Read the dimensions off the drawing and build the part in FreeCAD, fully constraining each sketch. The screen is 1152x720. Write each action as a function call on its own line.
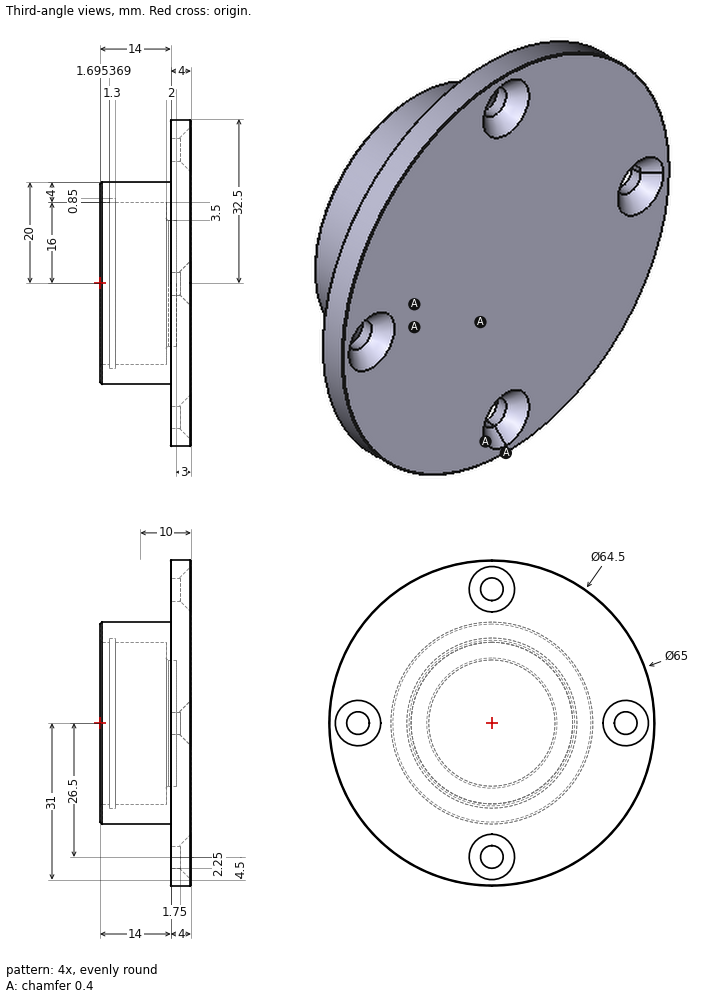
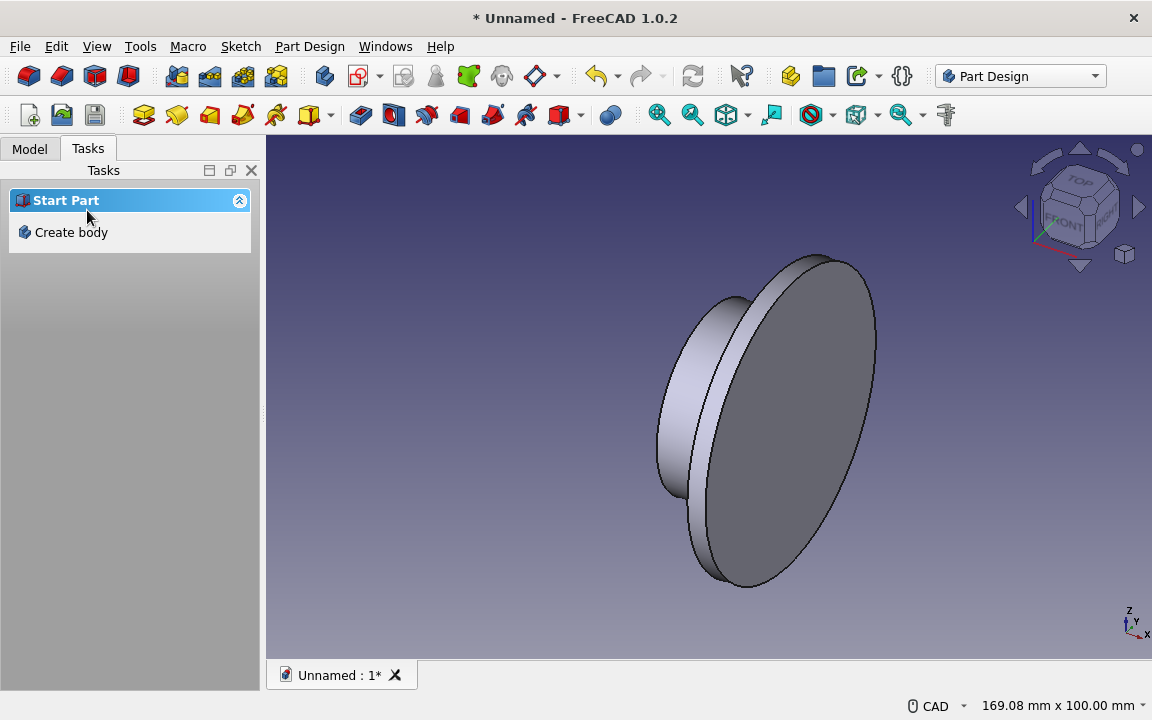
click(358, 76)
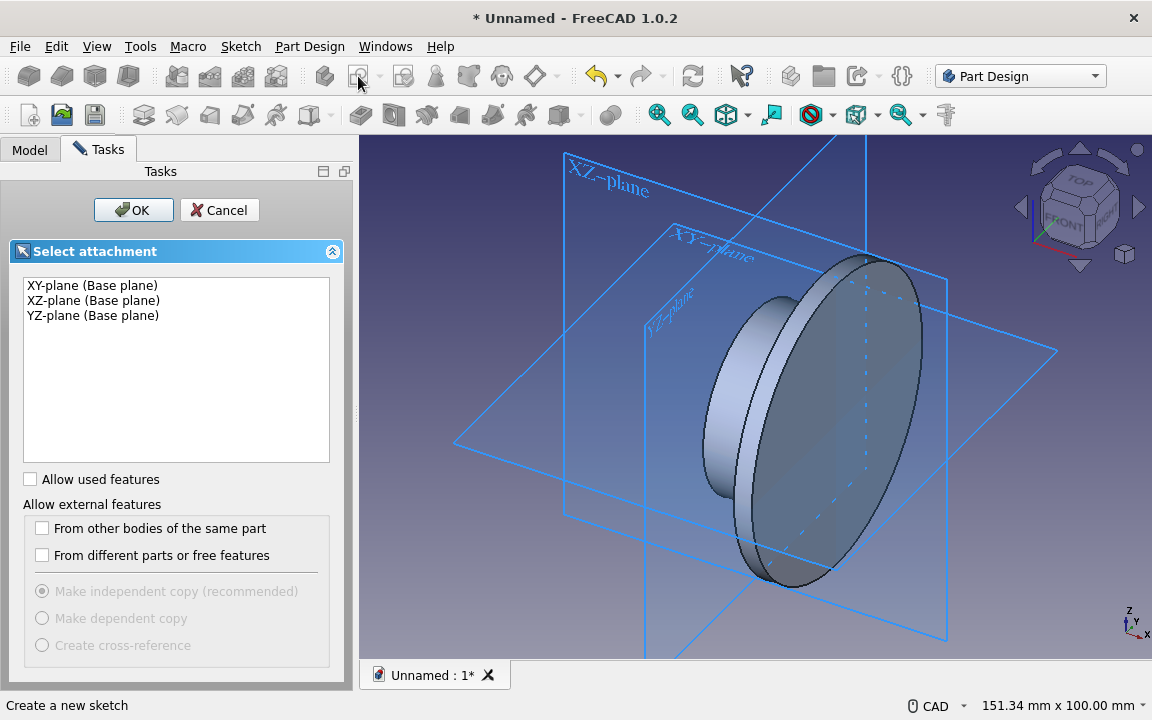
click(84, 300)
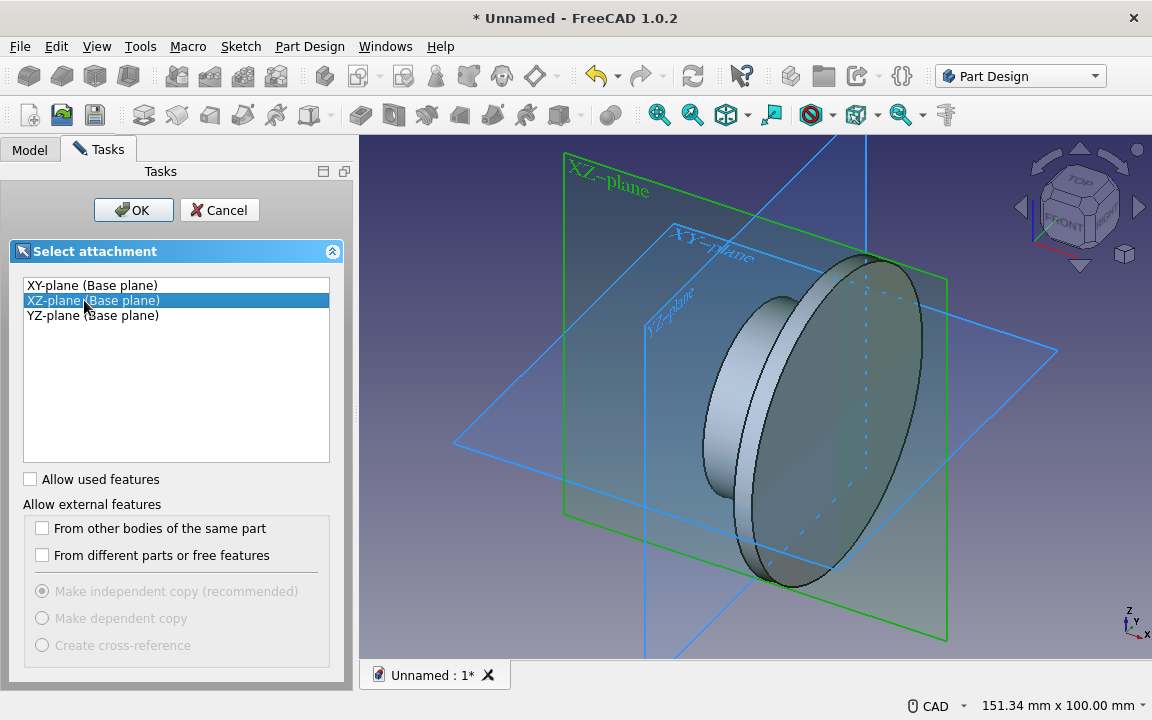
click(134, 210)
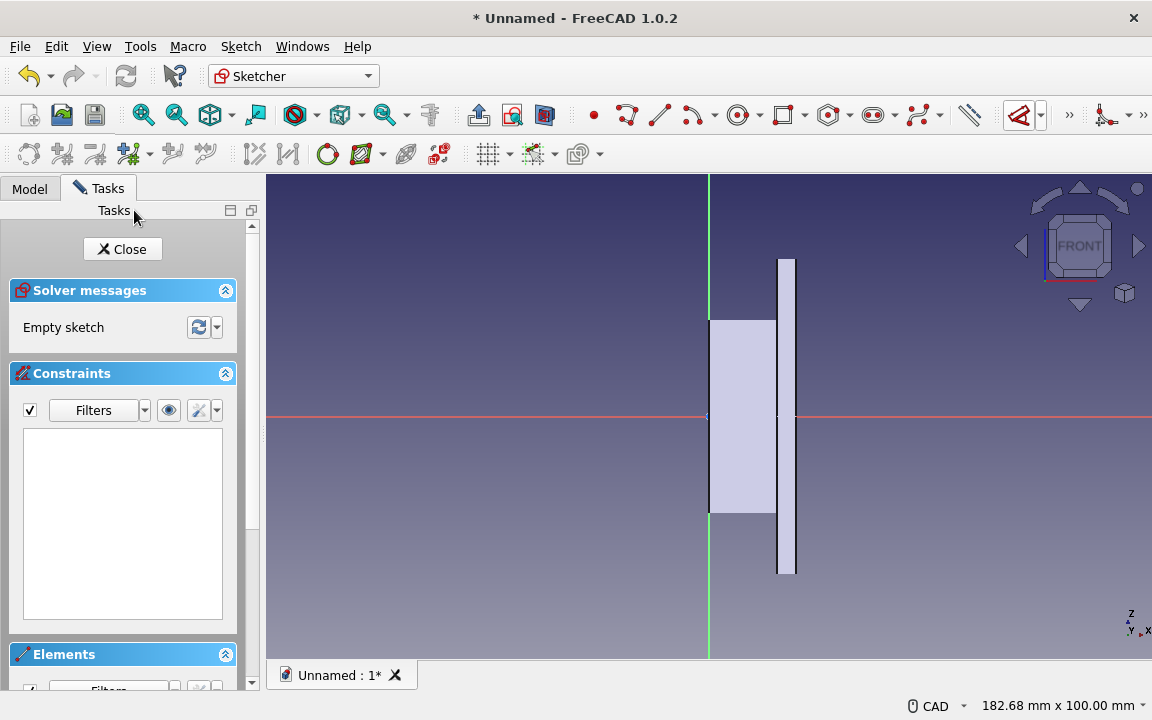
click(545, 116)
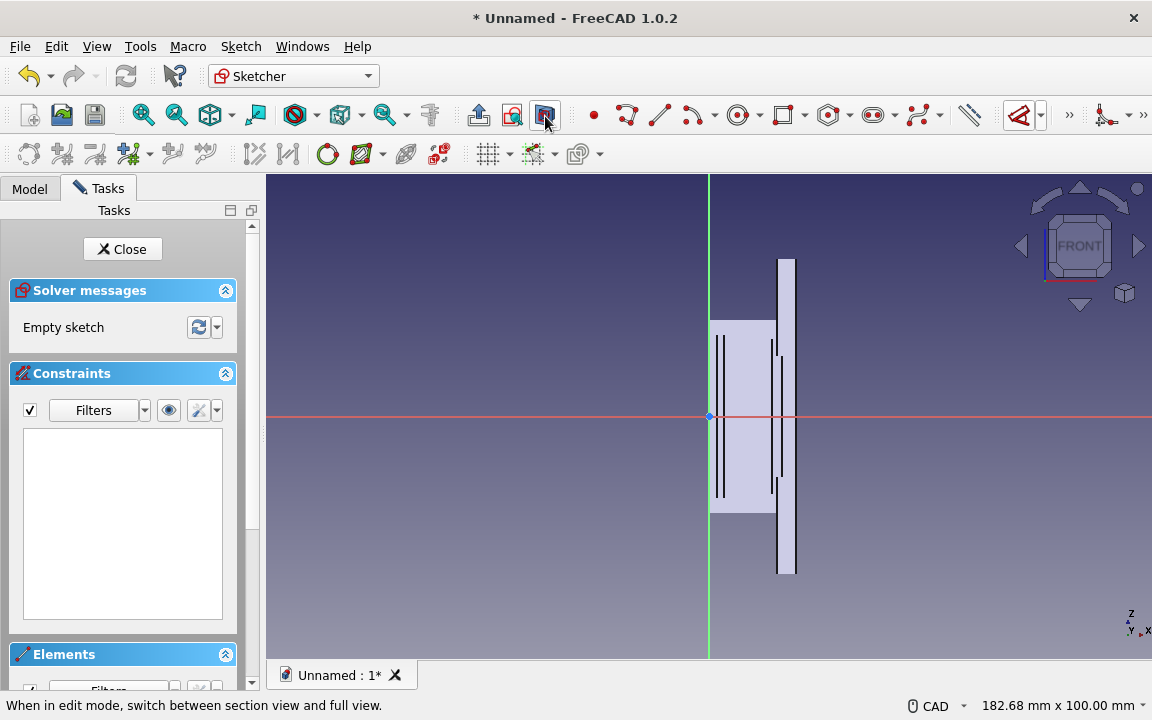
scroll(803, 567, up, 13)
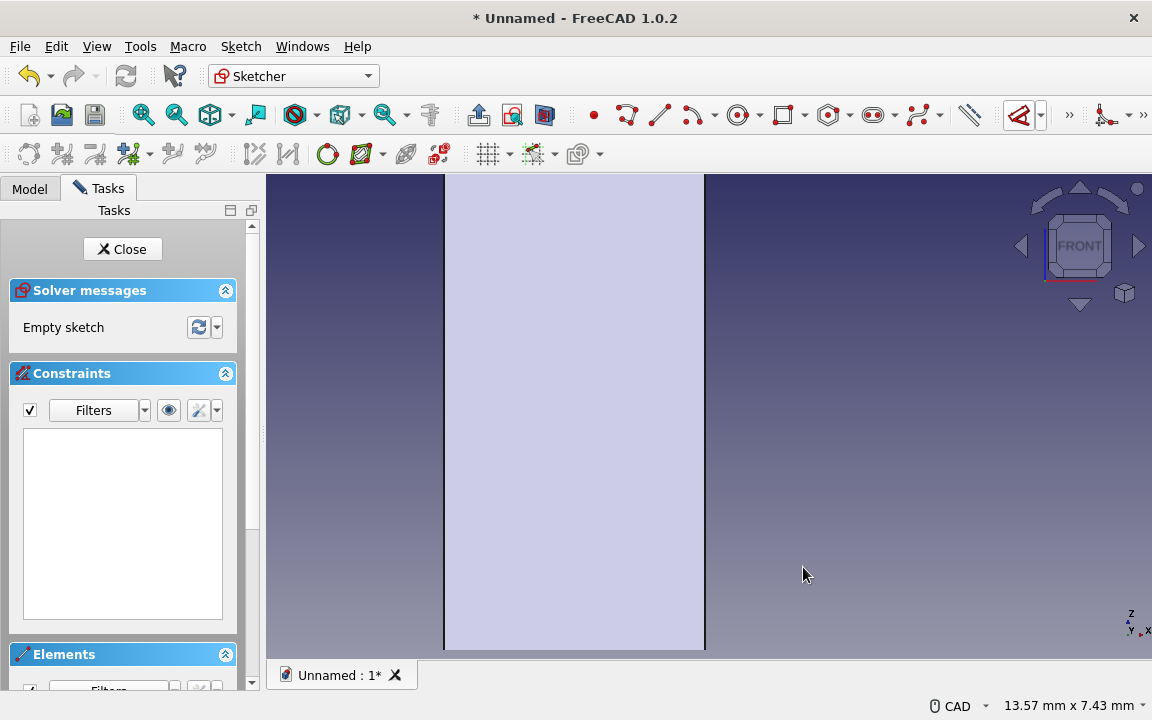
click(627, 116)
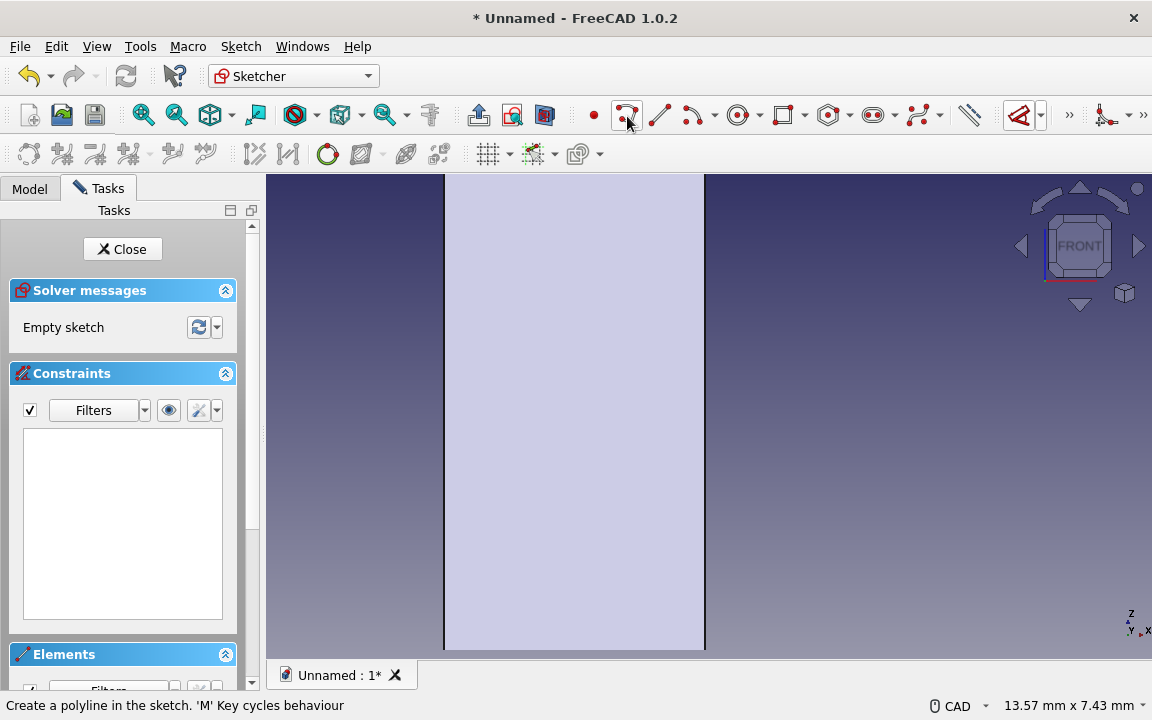
click(444, 261)
click(705, 261)
click(705, 555)
click(558, 408)
click(444, 408)
click(444, 262)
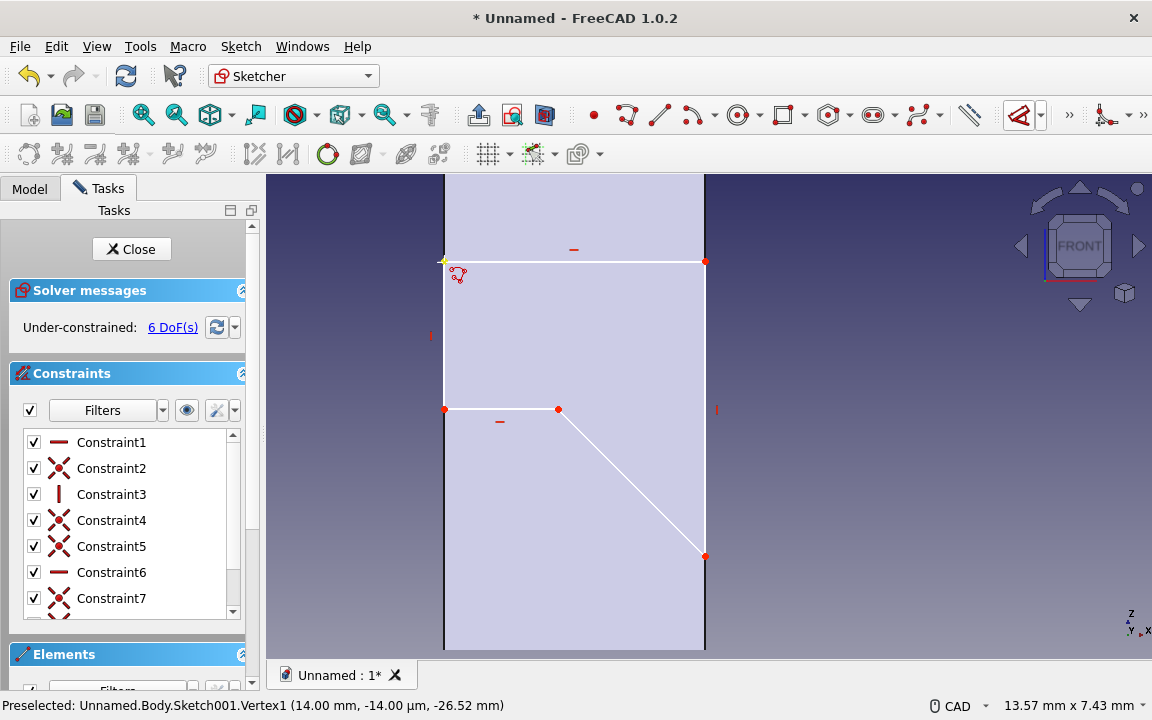
click(660, 116)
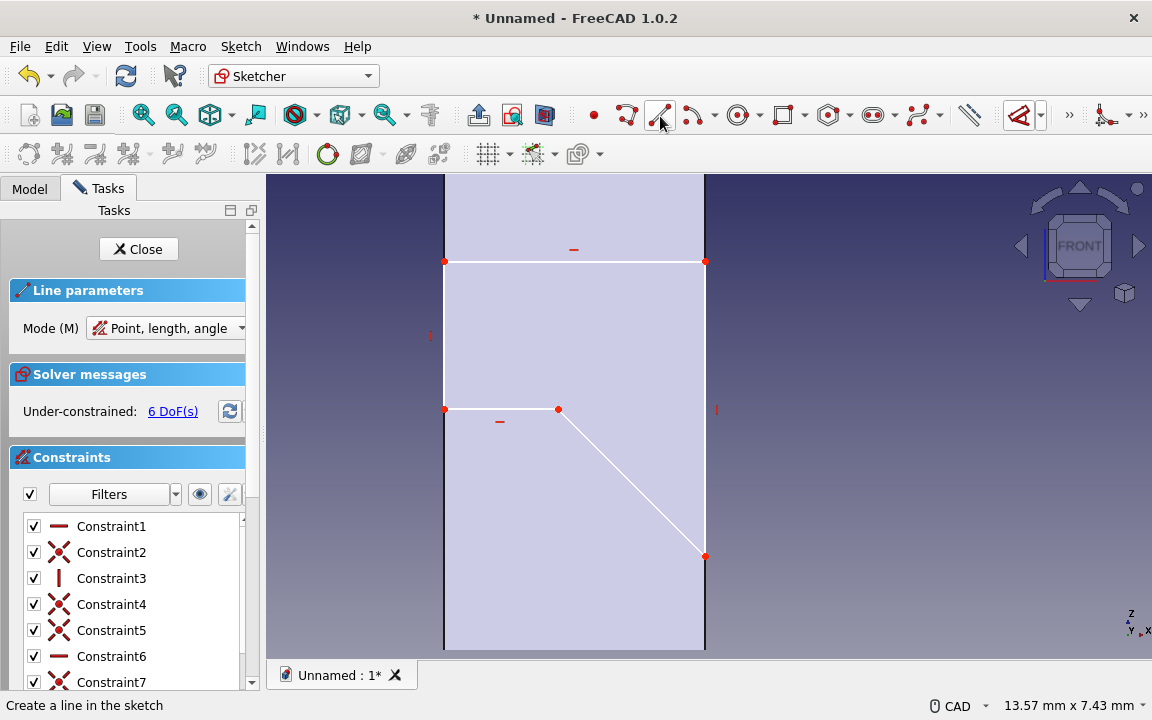
click(731, 261)
click(810, 261)
key(Escape)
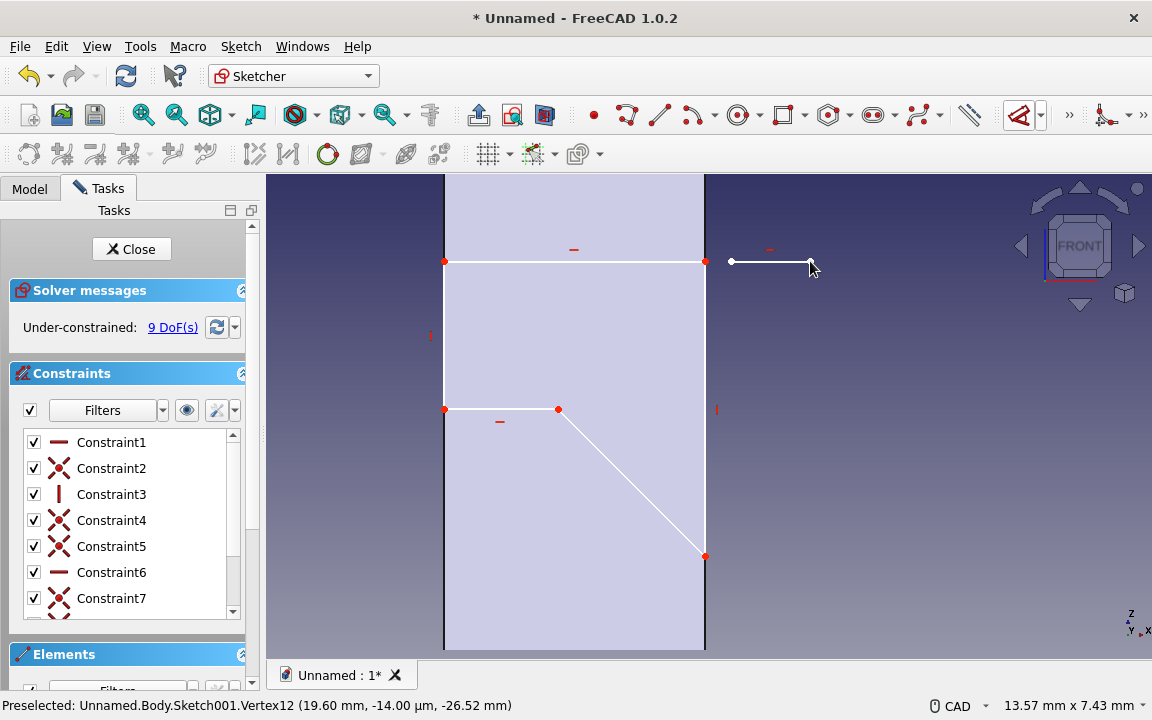
click(755, 262)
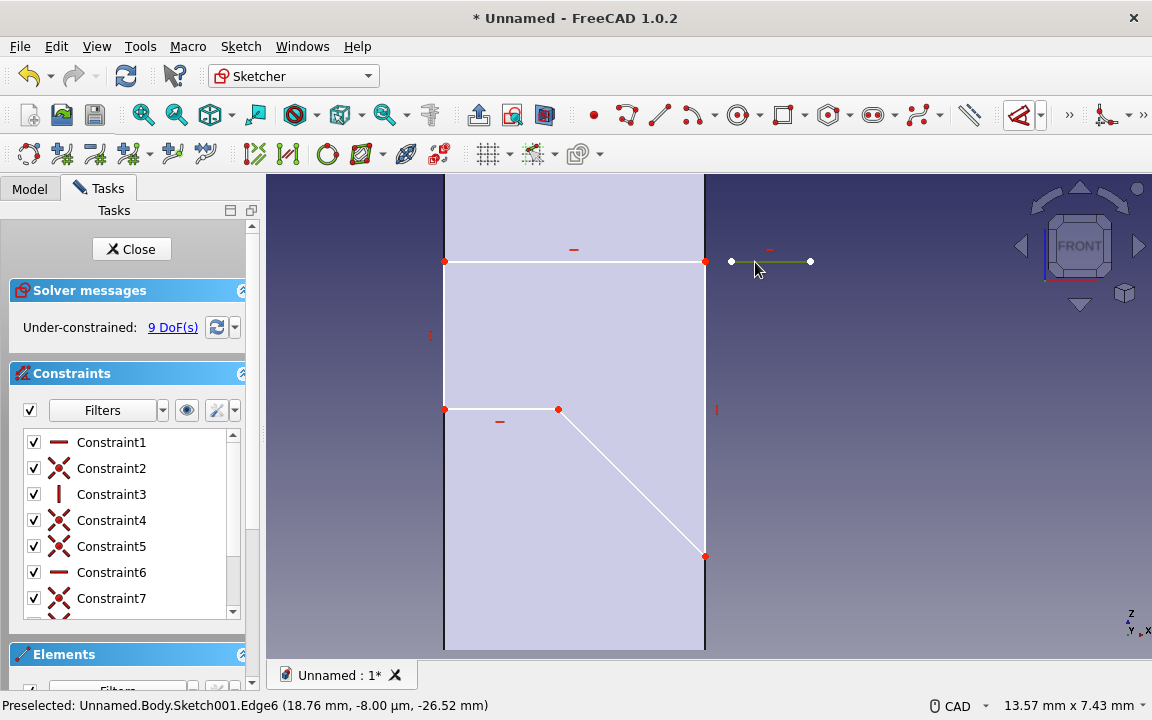
click(970, 116)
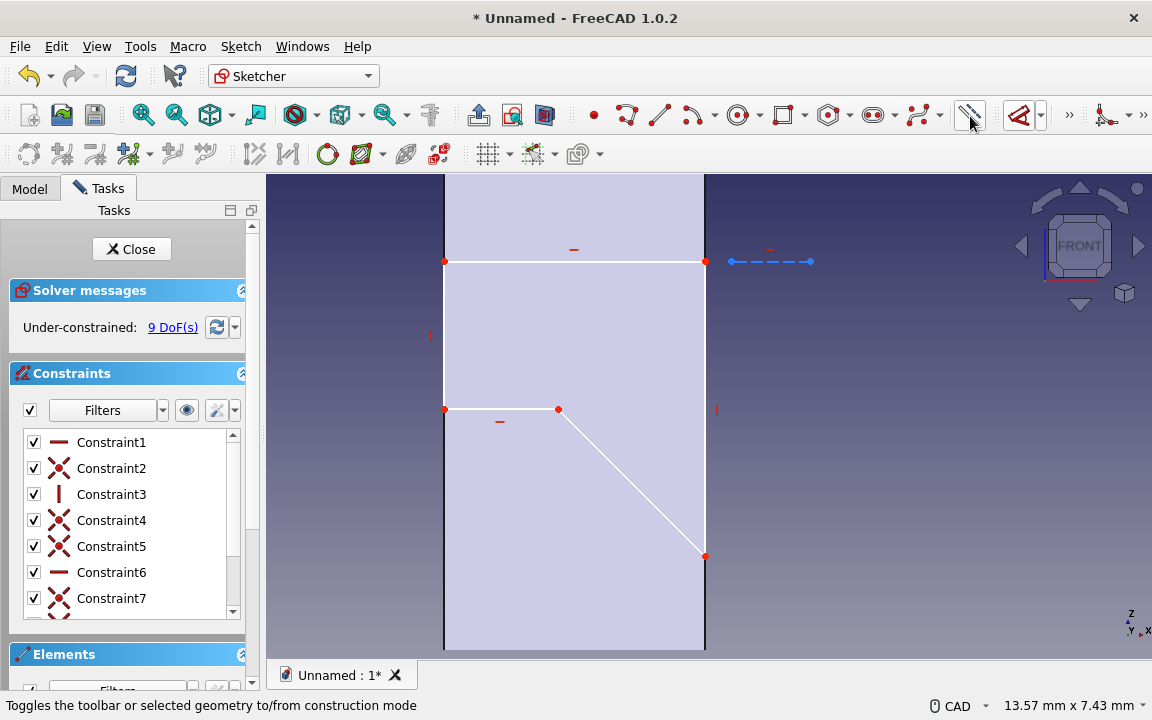
click(522, 262)